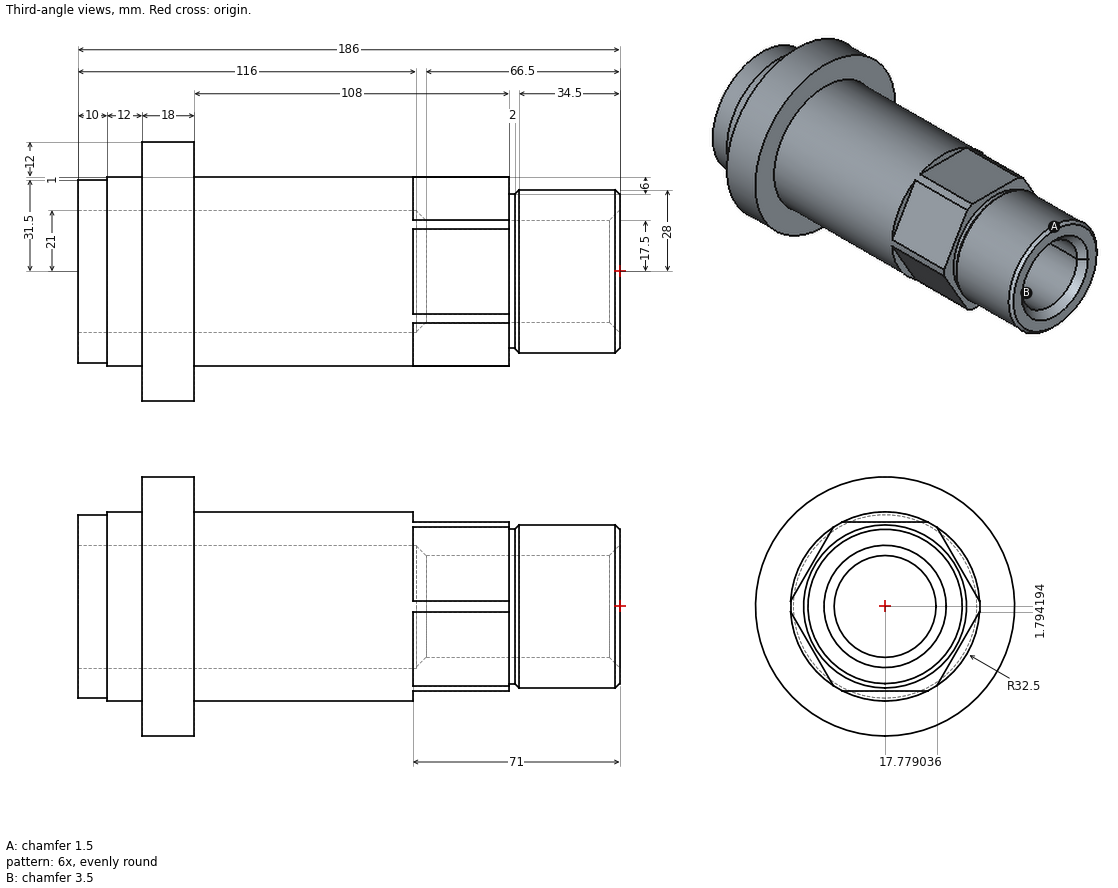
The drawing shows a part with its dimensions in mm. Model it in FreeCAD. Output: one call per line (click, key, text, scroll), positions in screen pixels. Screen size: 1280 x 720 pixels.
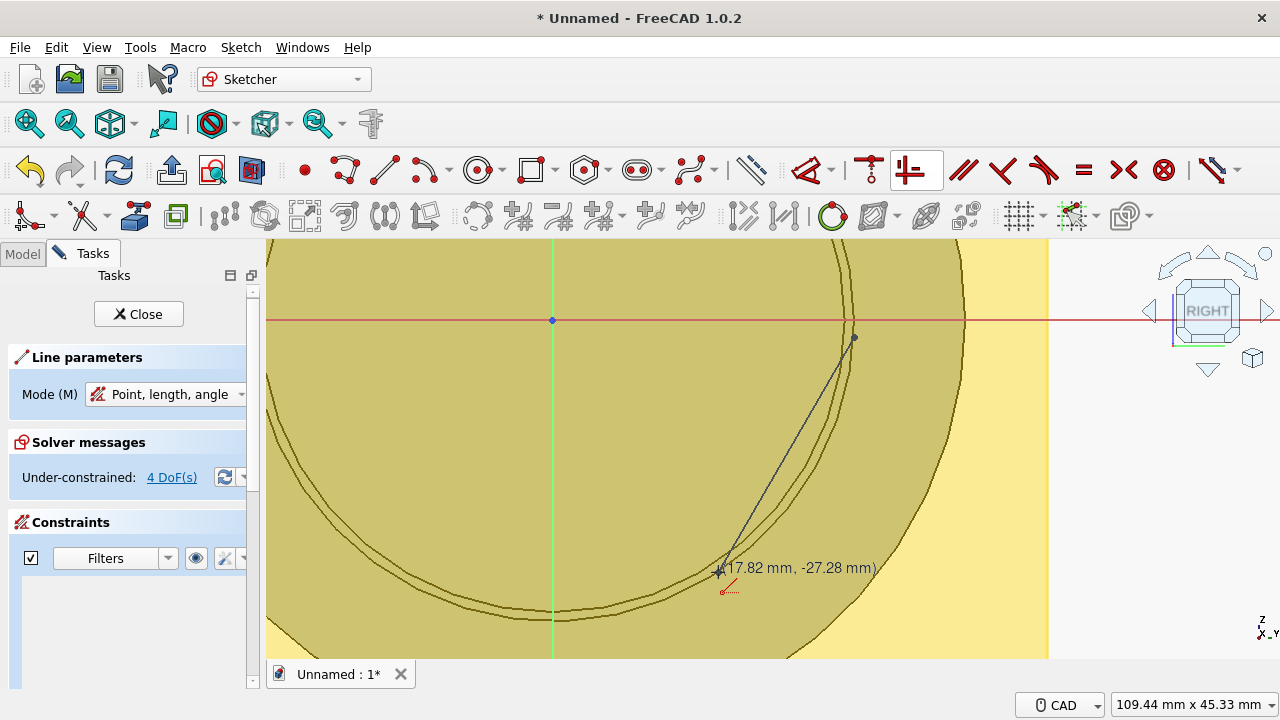
click(452, 170)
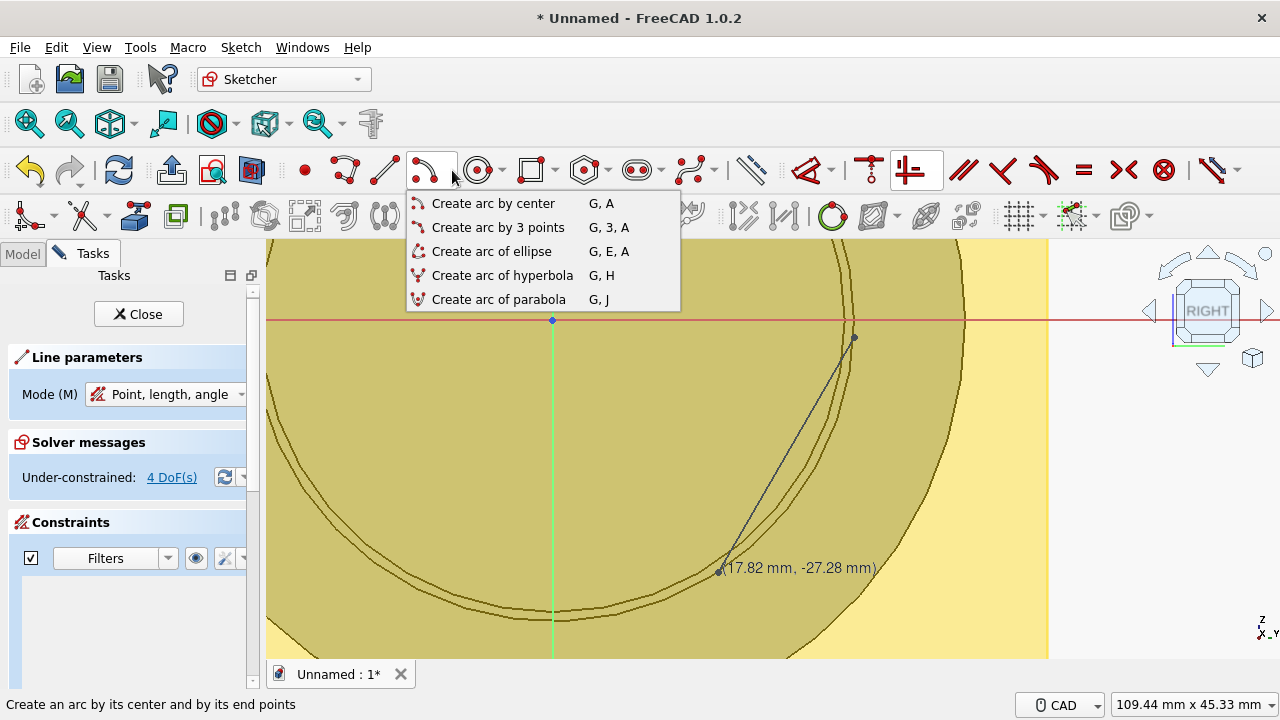
click(544, 227)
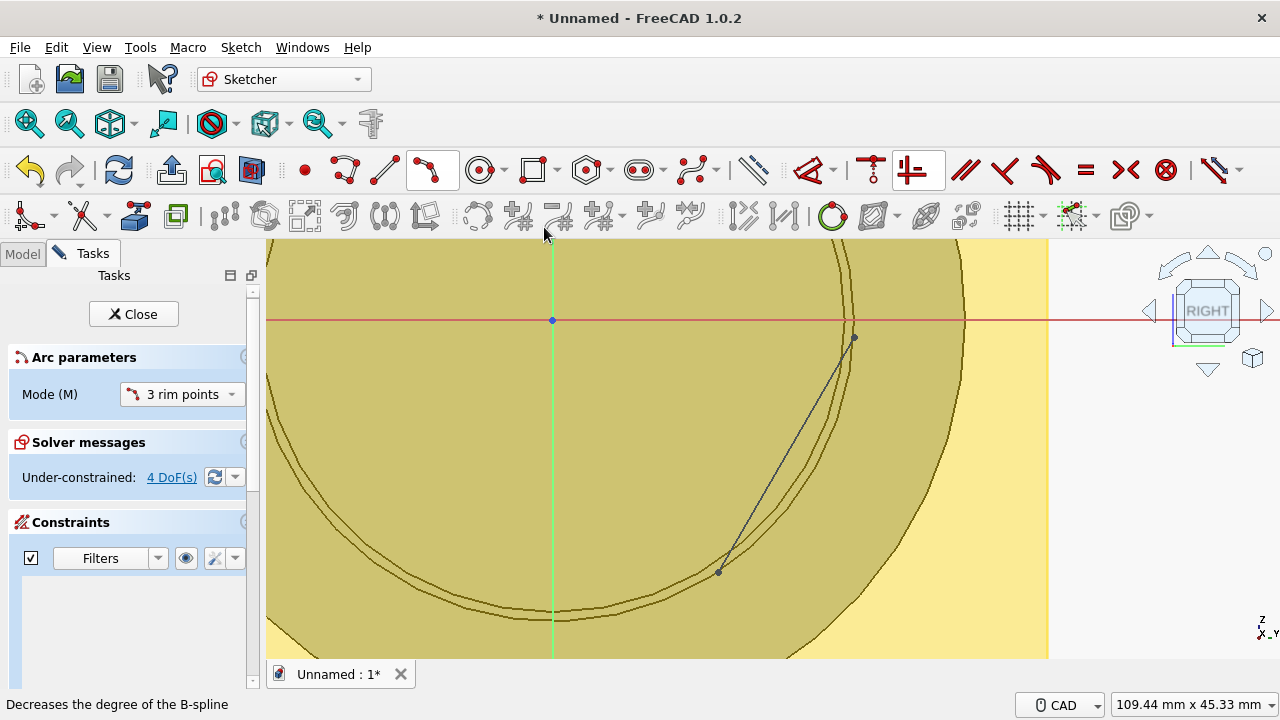
click(718, 573)
click(854, 338)
click(814, 471)
key(Escape)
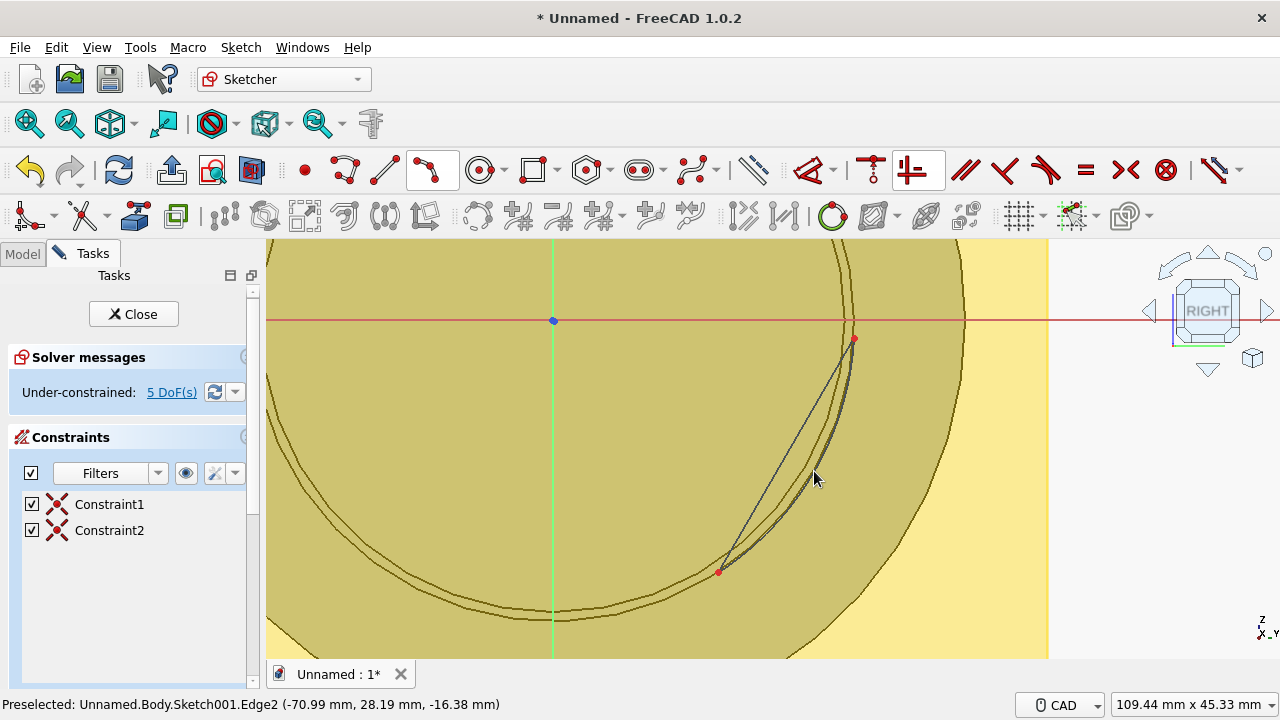
drag(543, 310, 565, 332)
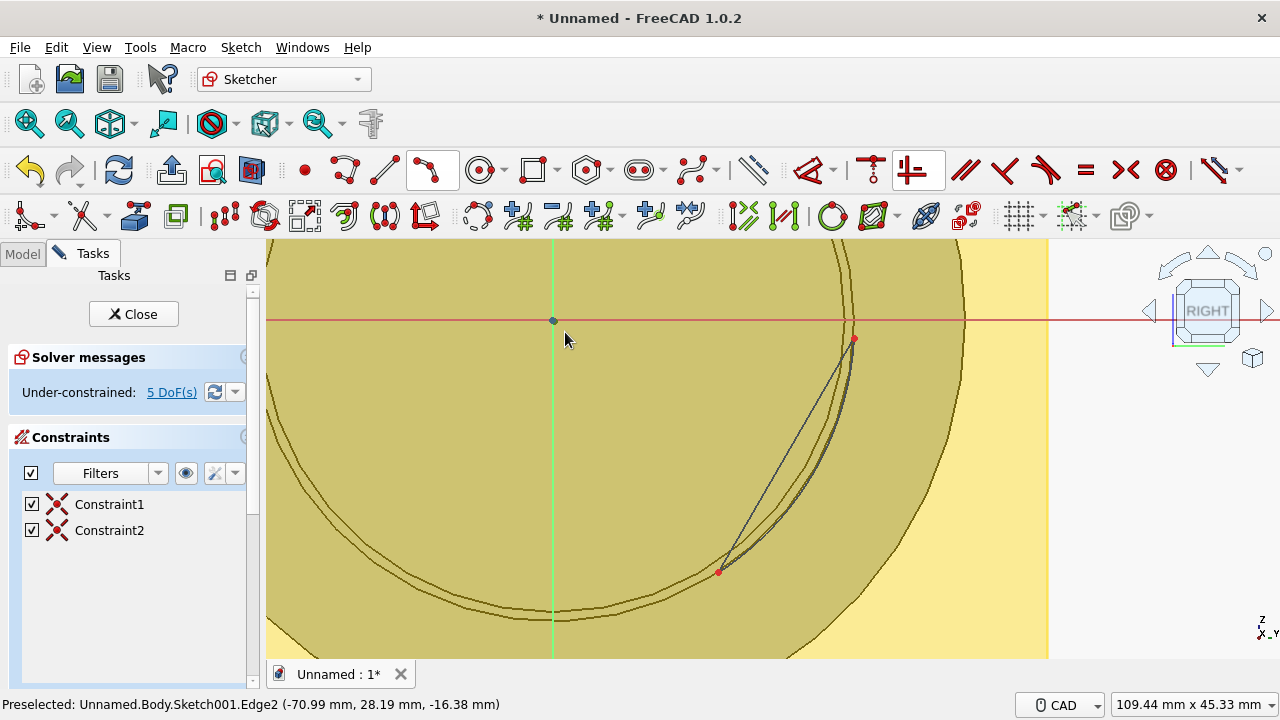
click(872, 170)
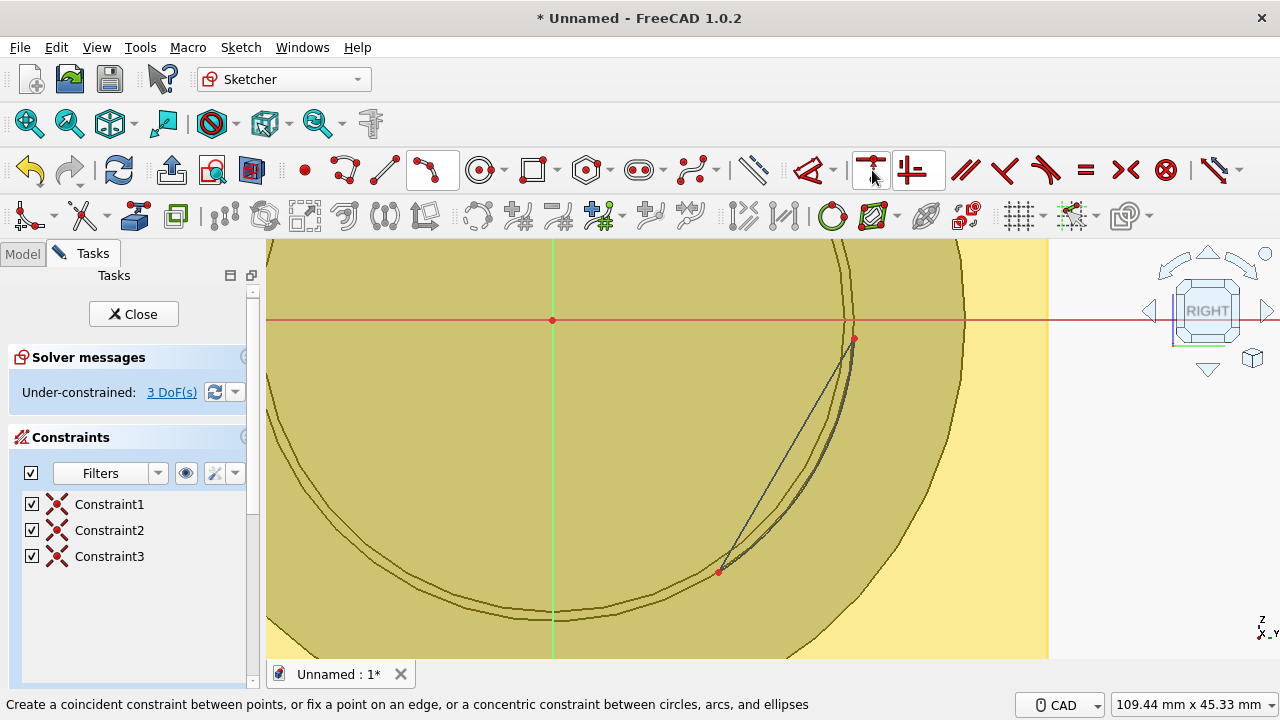
click(808, 170)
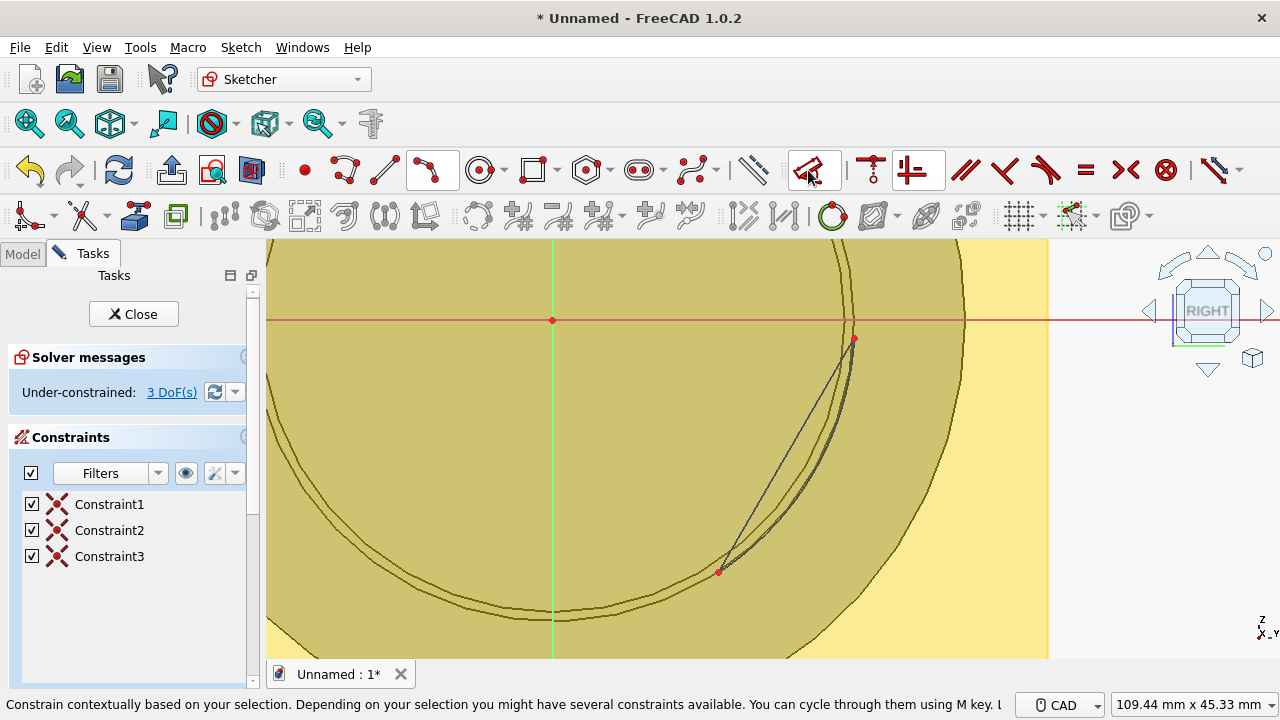
click(781, 518)
click(805, 539)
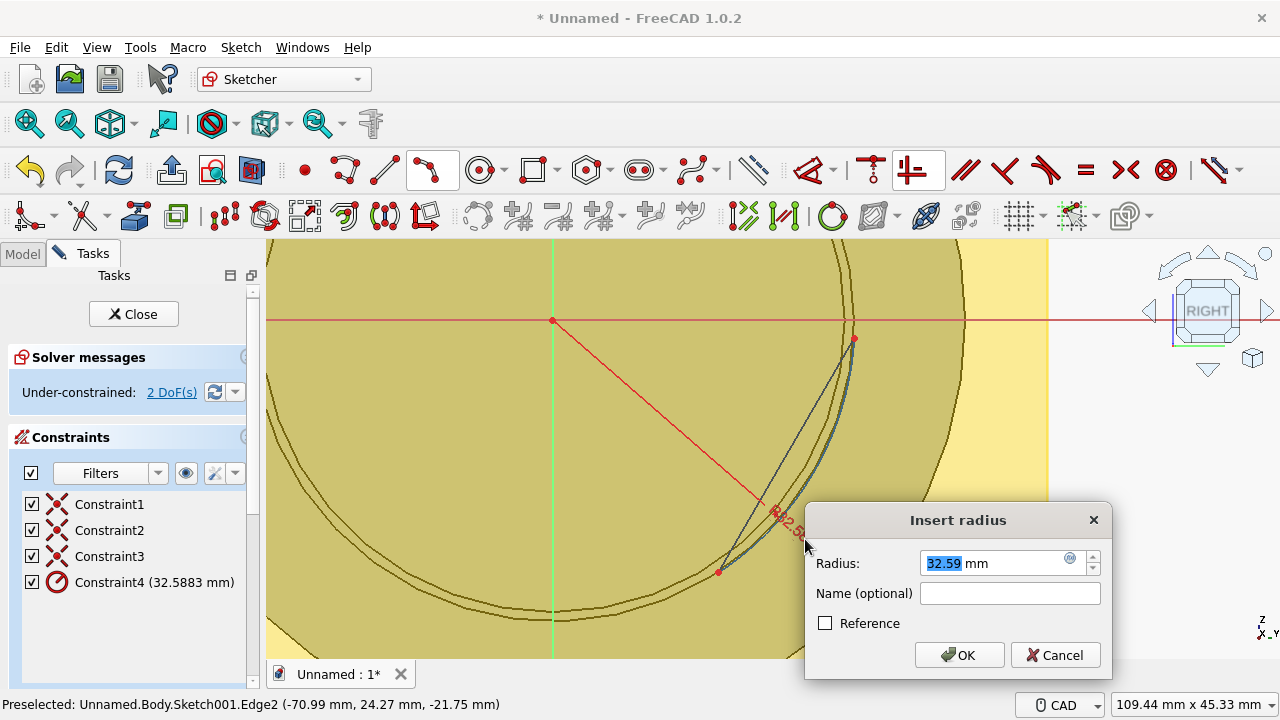
text(32.5)
key(Return)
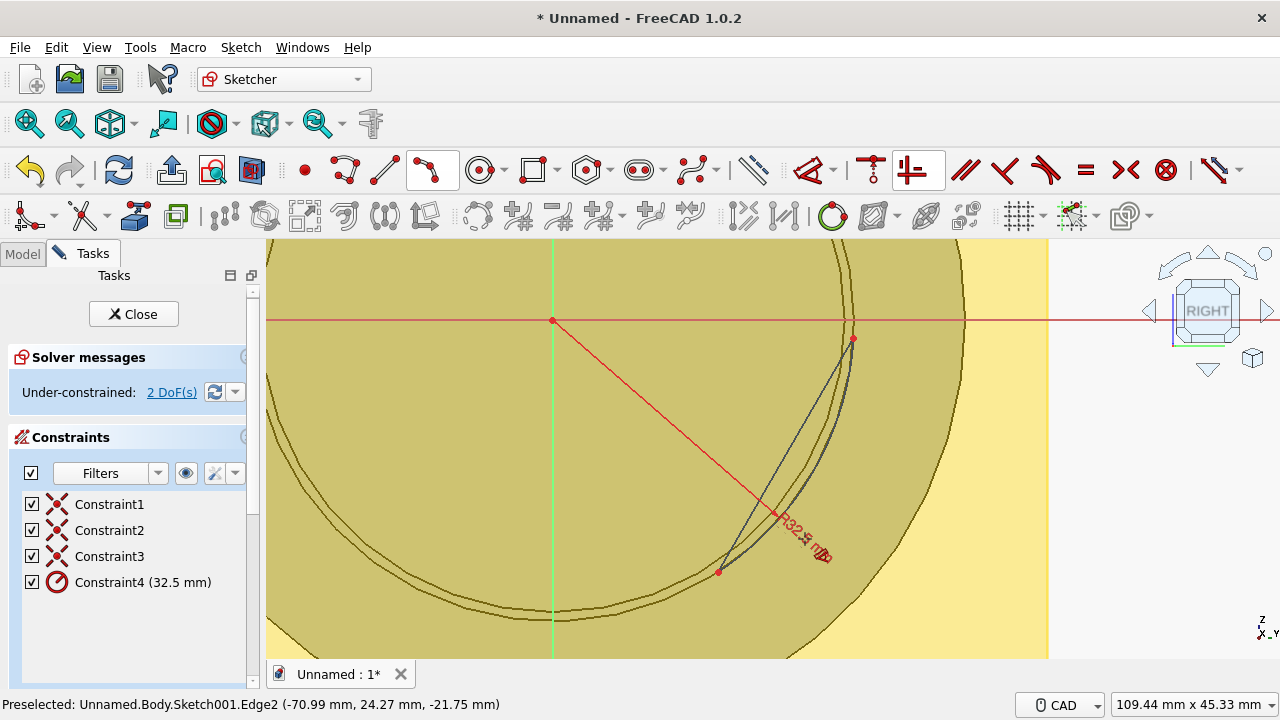
scroll(853, 338, up, 5)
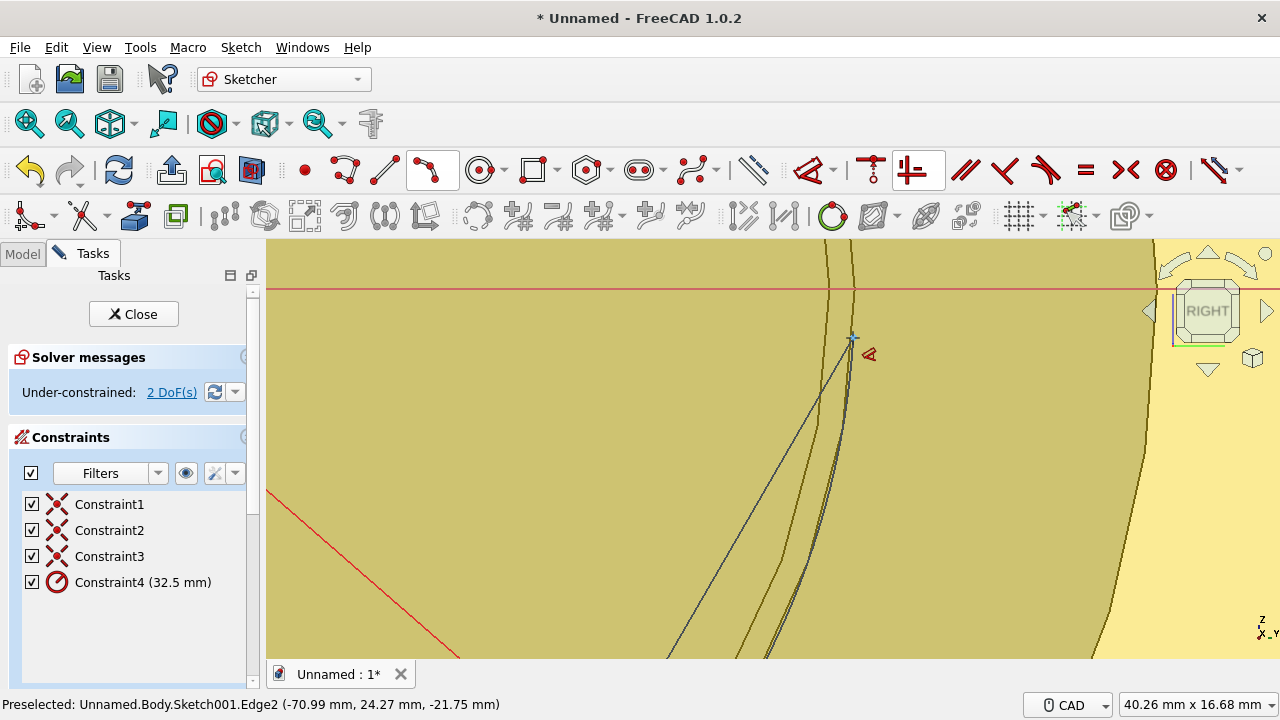
click(853, 338)
click(887, 313)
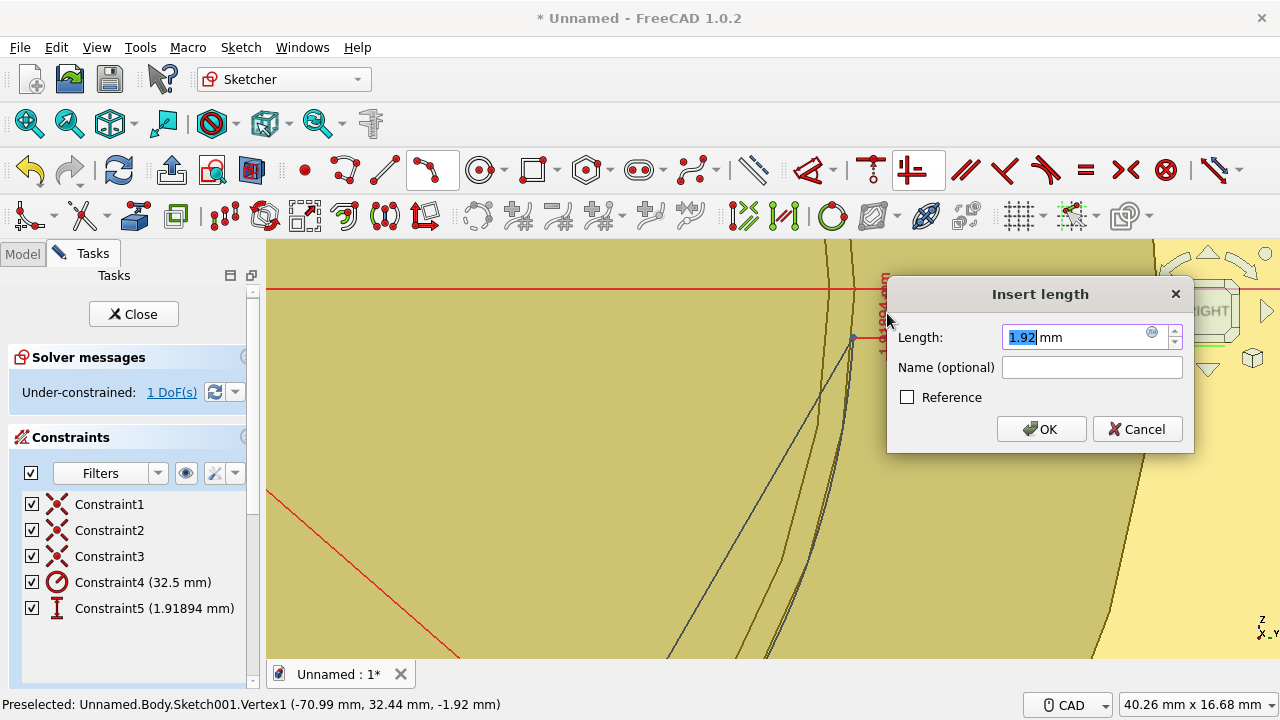
text(1.794194)
key(Return)